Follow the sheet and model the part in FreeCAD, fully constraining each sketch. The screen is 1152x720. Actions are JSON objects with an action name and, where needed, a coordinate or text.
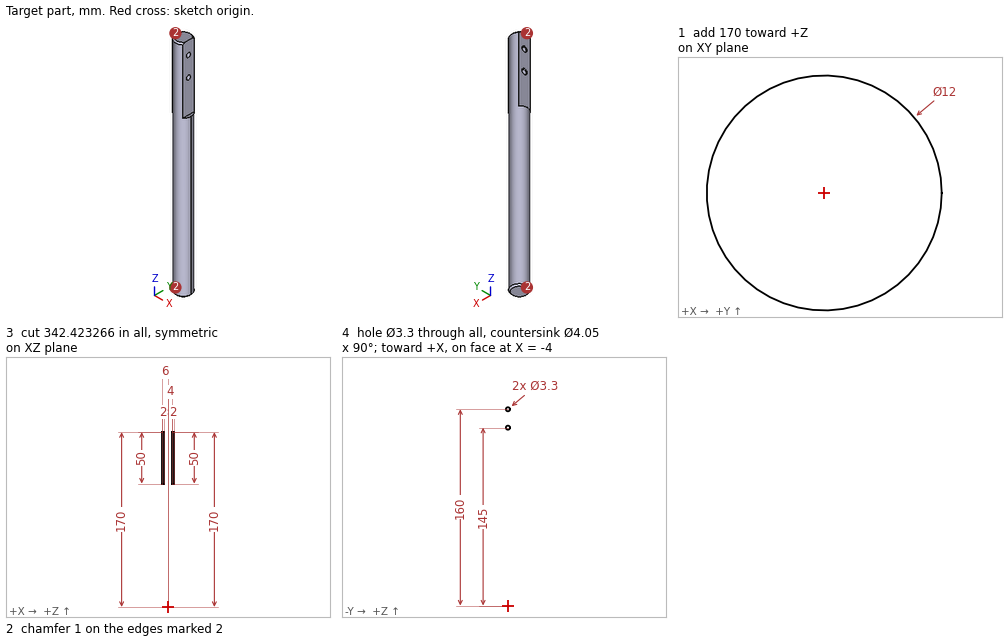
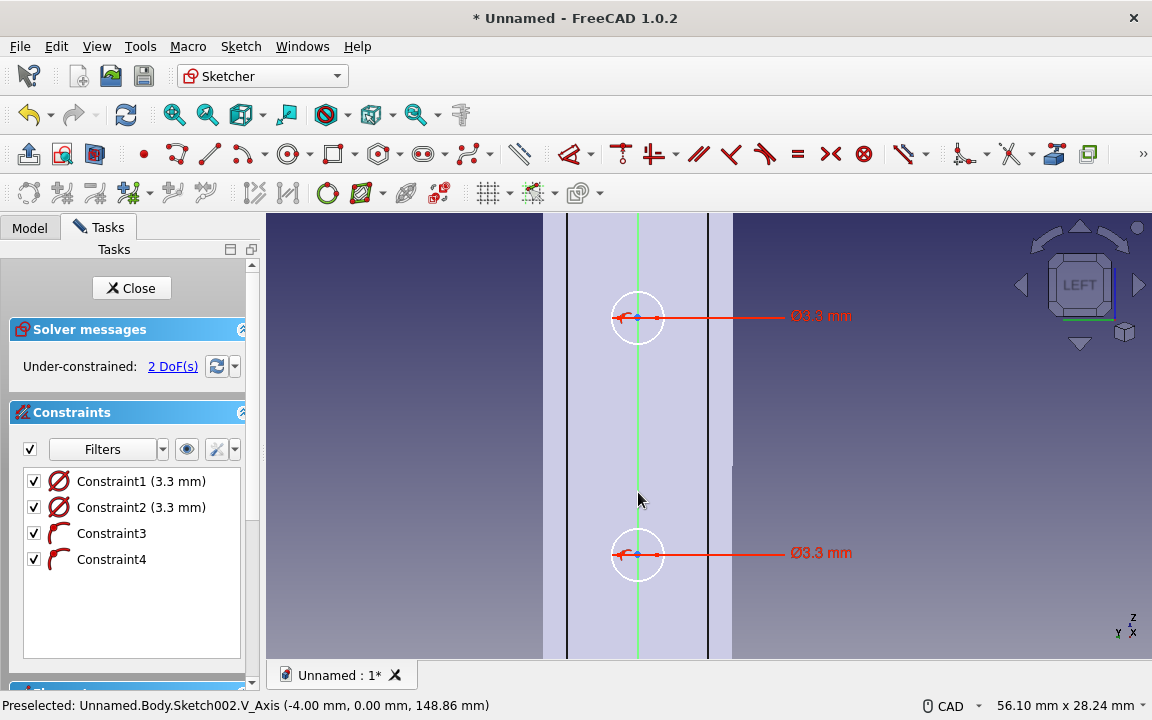
{"action": "key", "text": "d"}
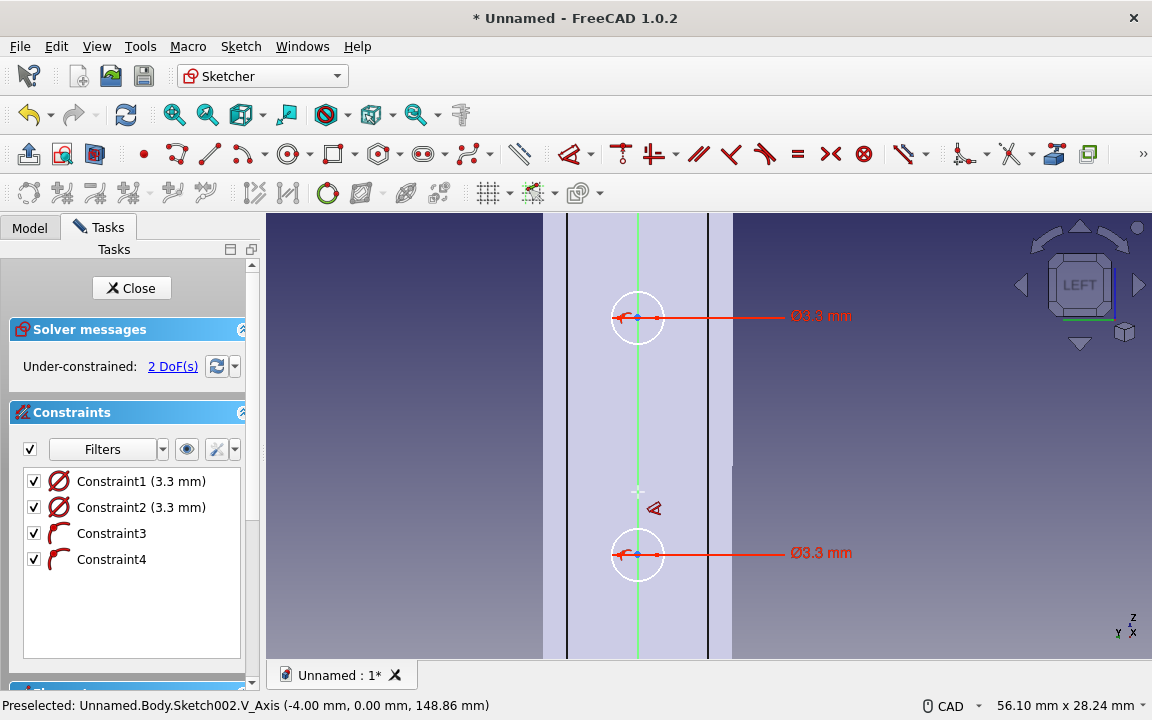
{"action": "left_click", "coordinate": [638, 318]}
{"action": "left_click", "coordinate": [672, 474]}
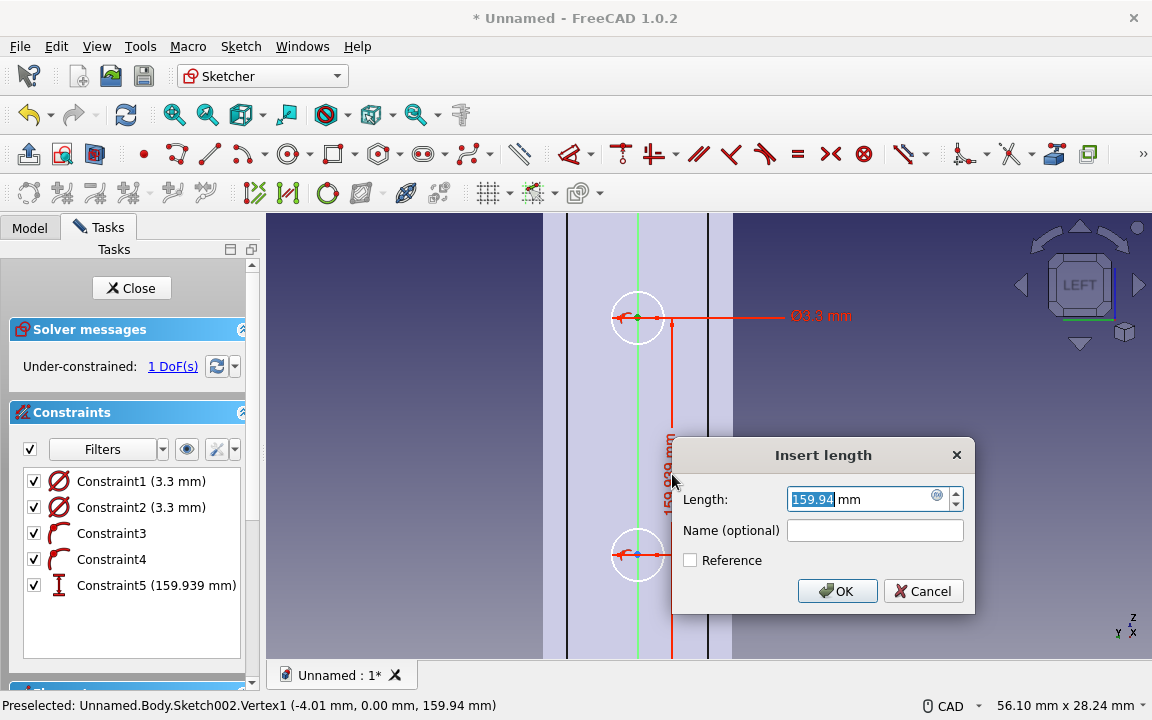
{"action": "type", "text": "160"}
{"action": "key", "text": "Return"}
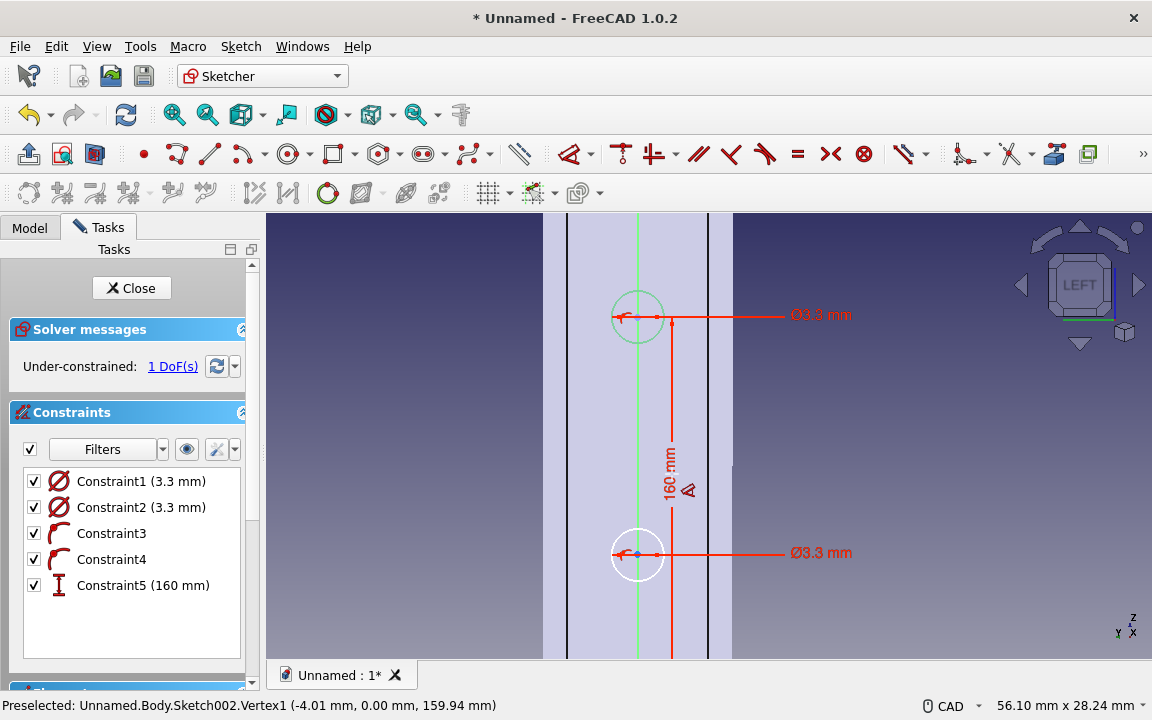
{"action": "left_click", "coordinate": [638, 555]}
{"action": "left_click", "coordinate": [672, 593]}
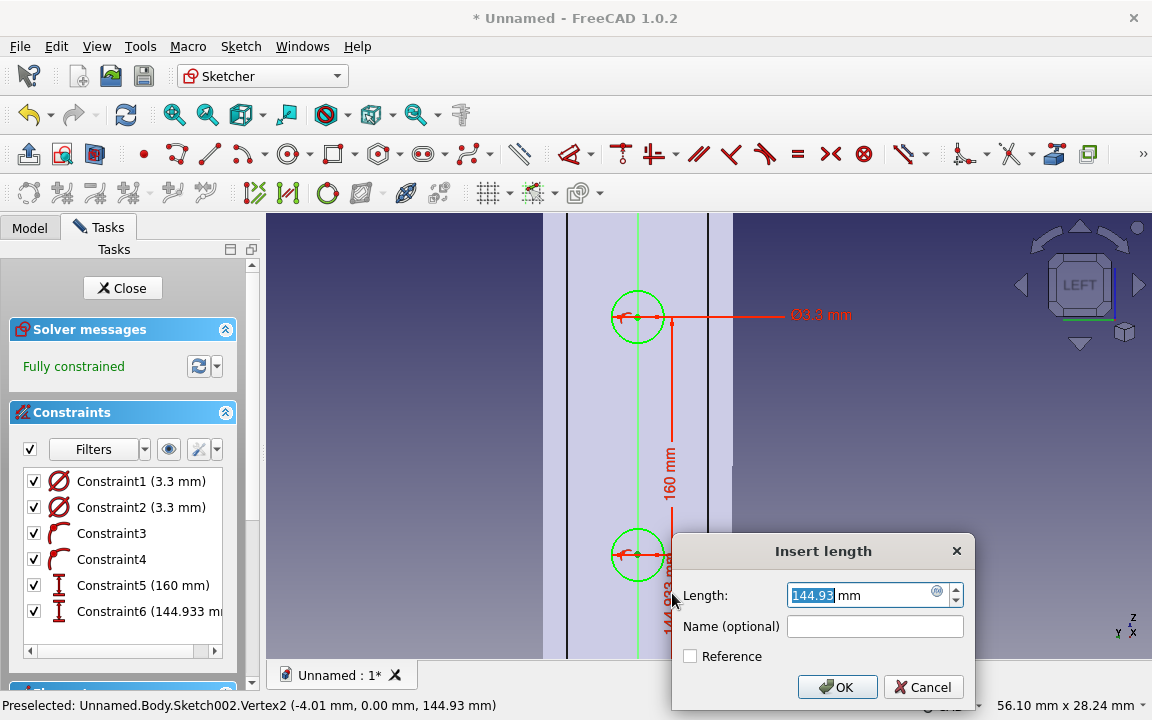
{"action": "type", "text": "145"}
{"action": "key", "text": "Return"}
{"action": "key", "text": "Escape"}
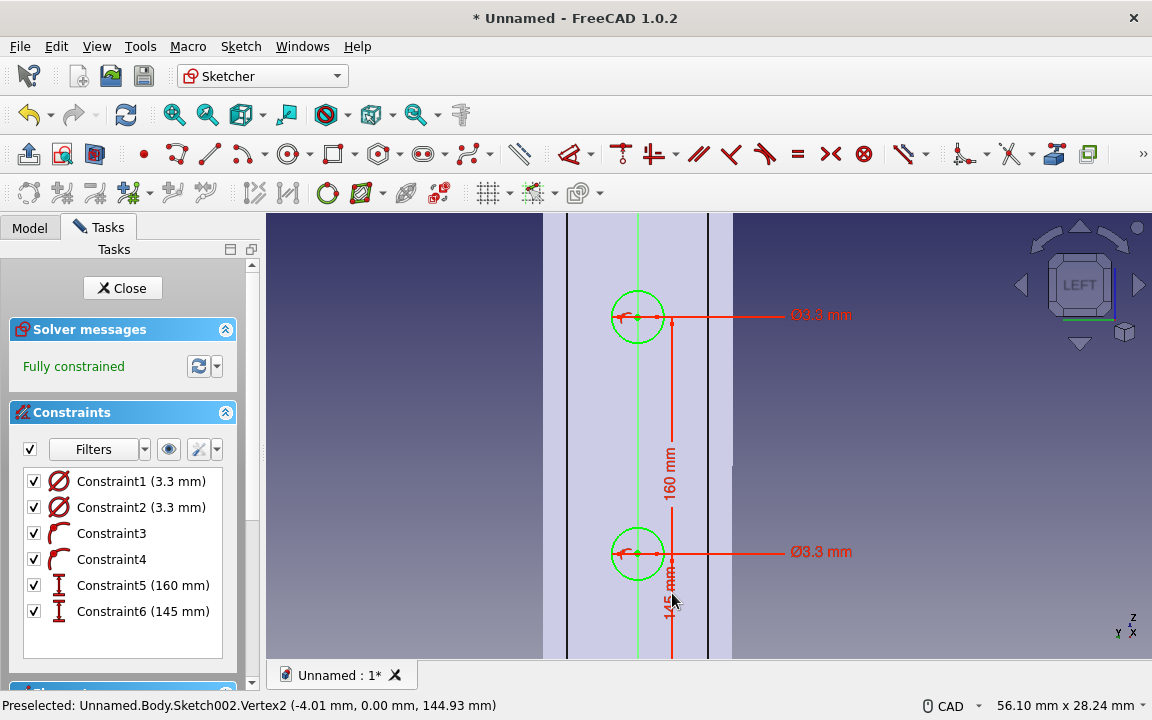
{"action": "left_click", "coordinate": [123, 288]}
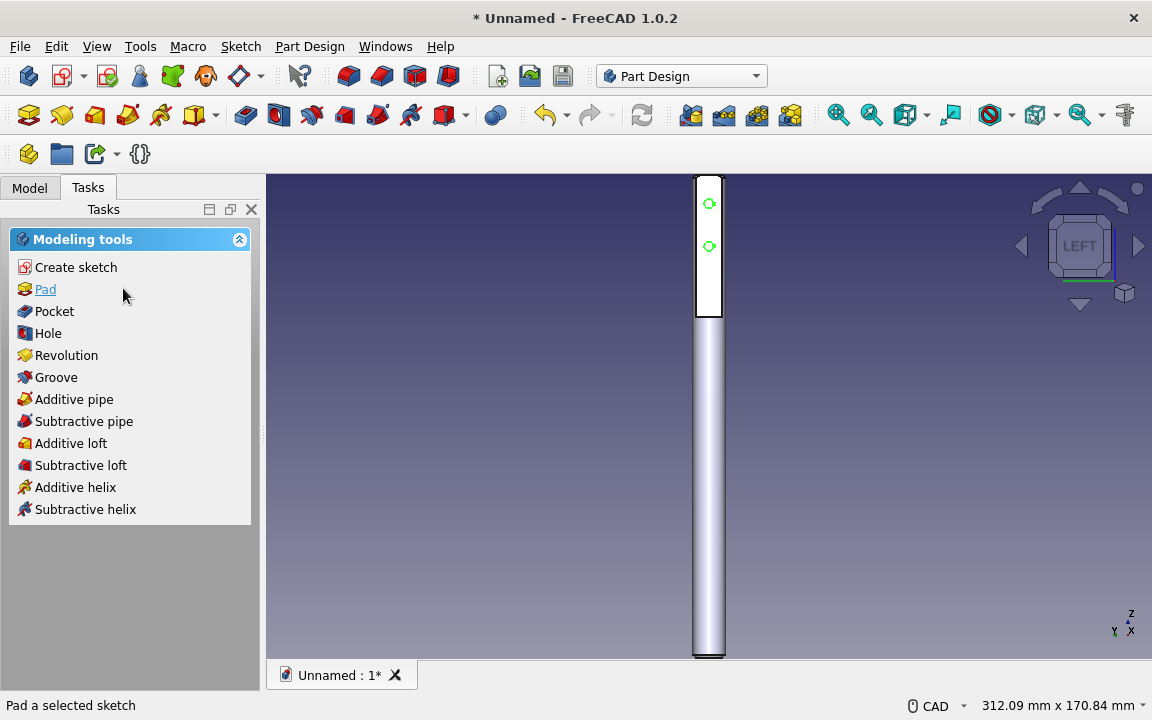
{"action": "left_click", "coordinate": [279, 116]}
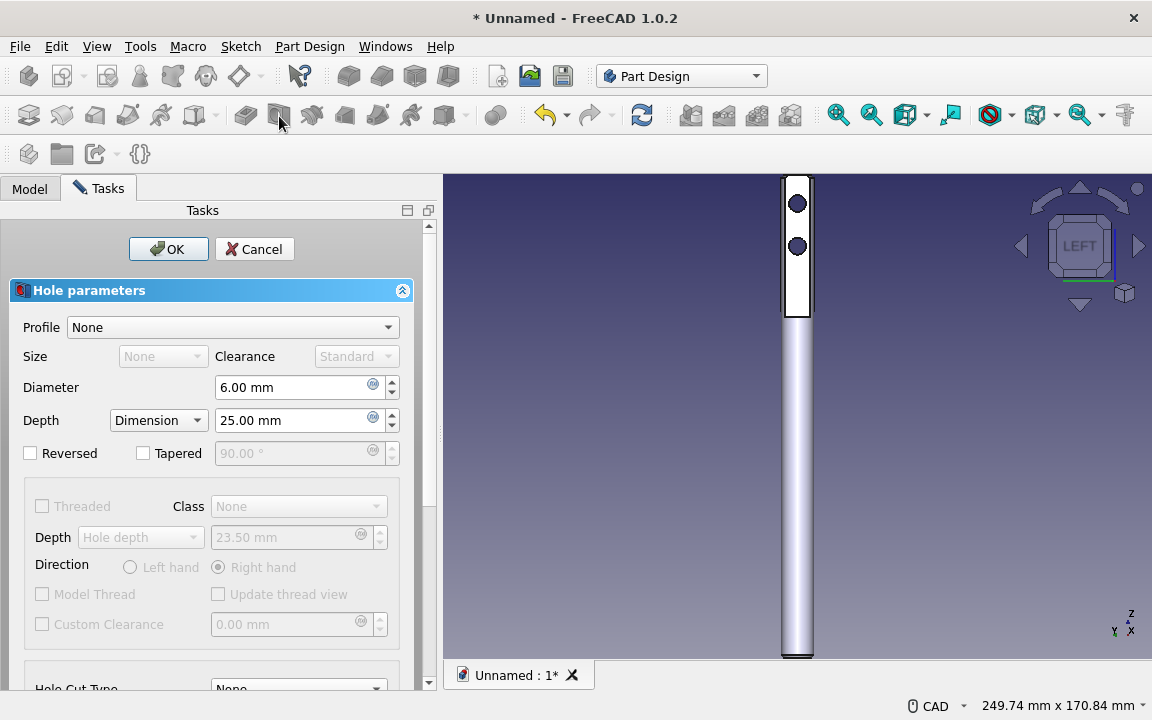
{"action": "triple_click", "coordinate": [300, 388]}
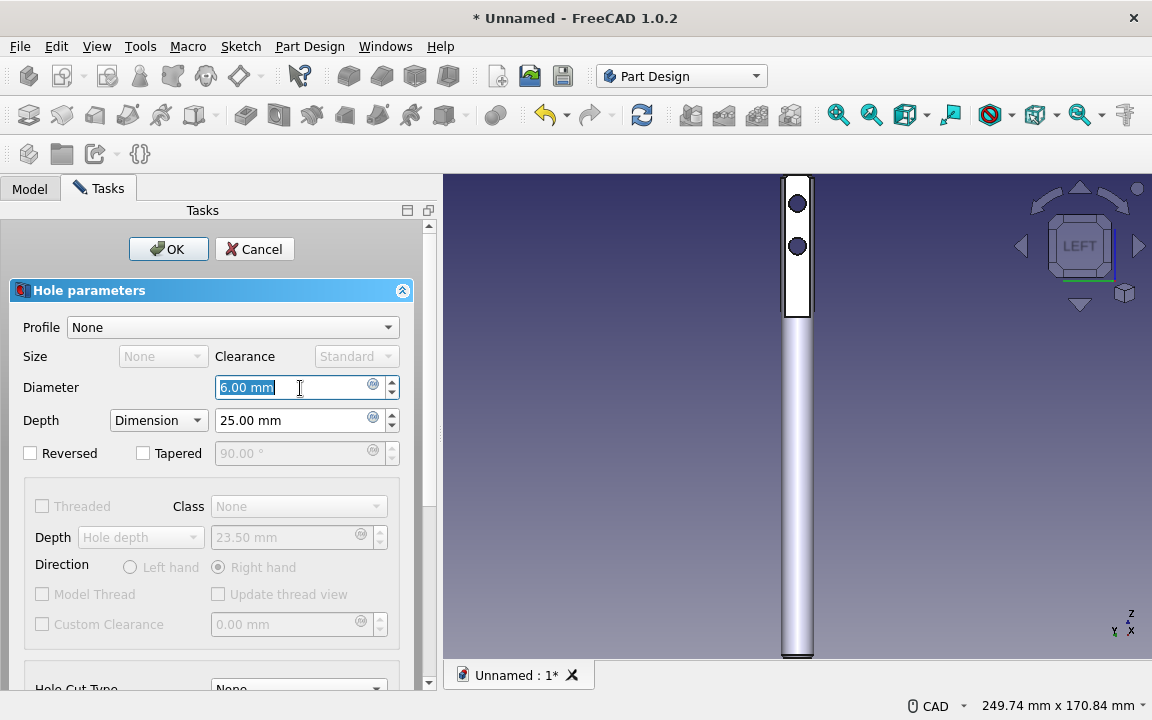
{"action": "type", "text": "3.3"}
{"action": "key", "text": "Tab"}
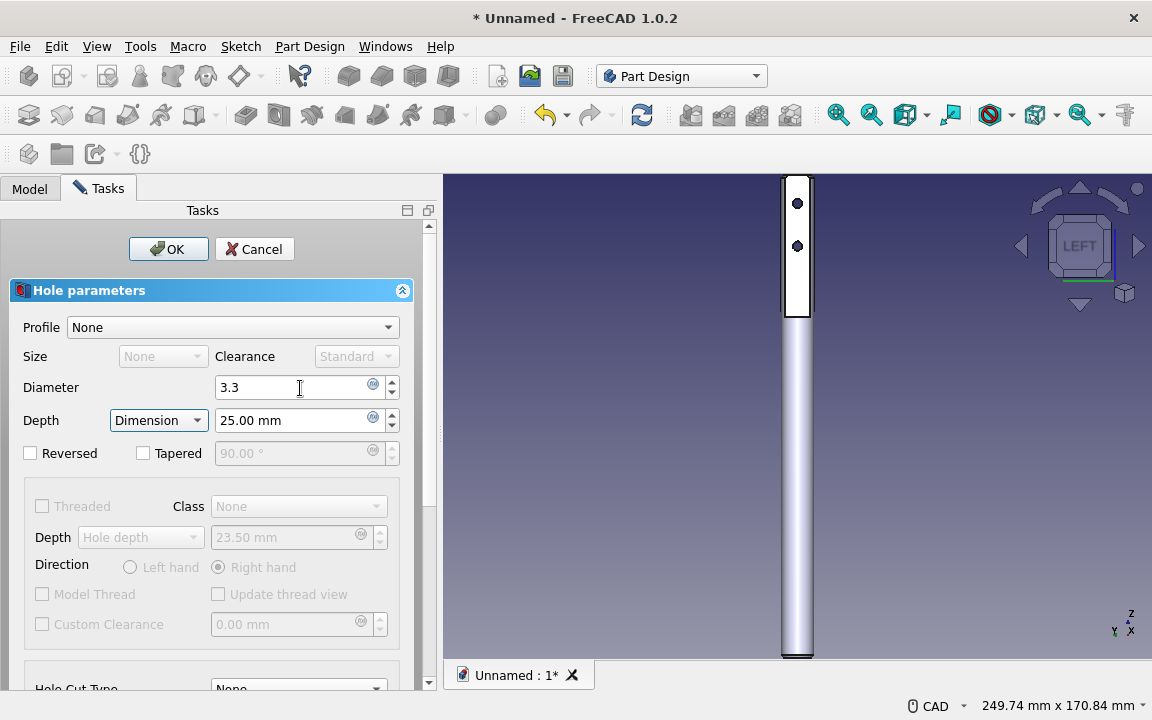
{"action": "left_click", "coordinate": [160, 420]}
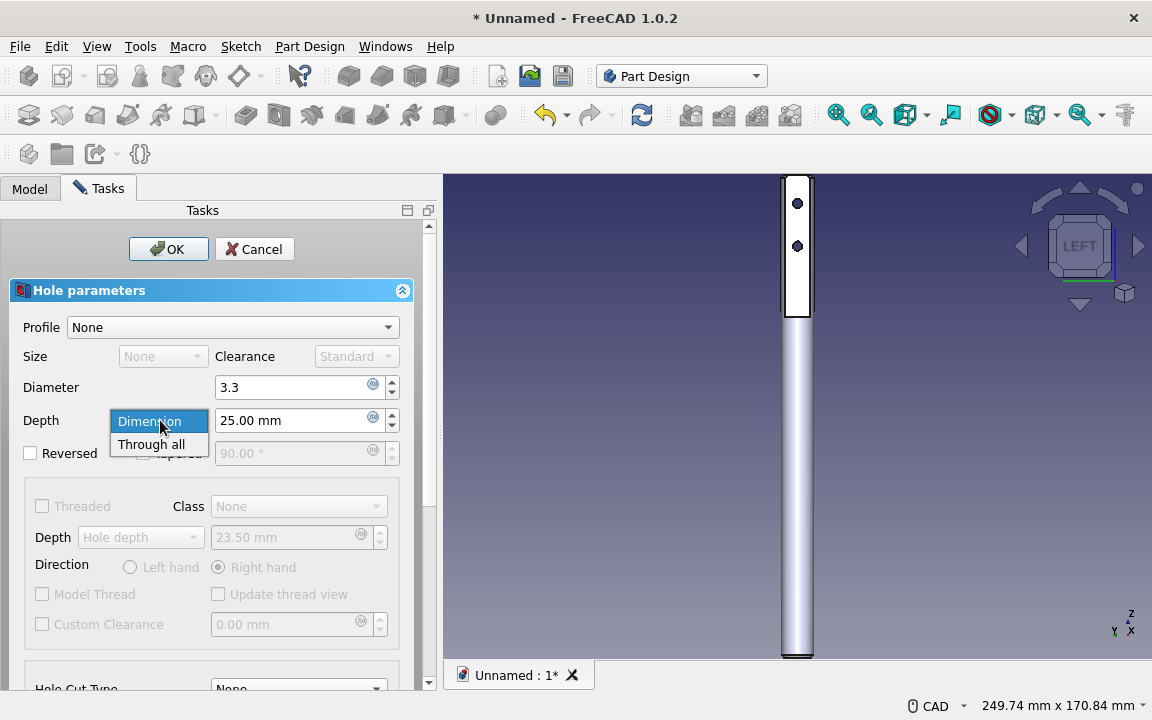
{"action": "left_click", "coordinate": [158, 444]}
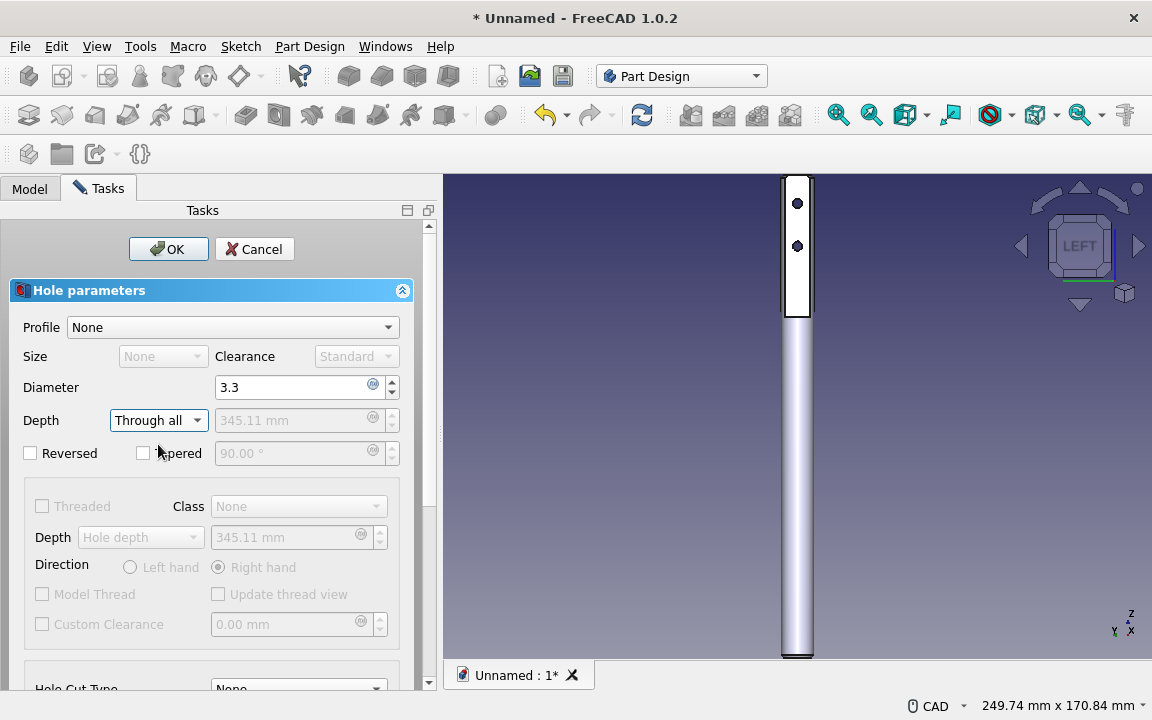
{"action": "scroll", "coordinate": [429, 455], "scroll_direction": "down", "scroll_amount": 2}